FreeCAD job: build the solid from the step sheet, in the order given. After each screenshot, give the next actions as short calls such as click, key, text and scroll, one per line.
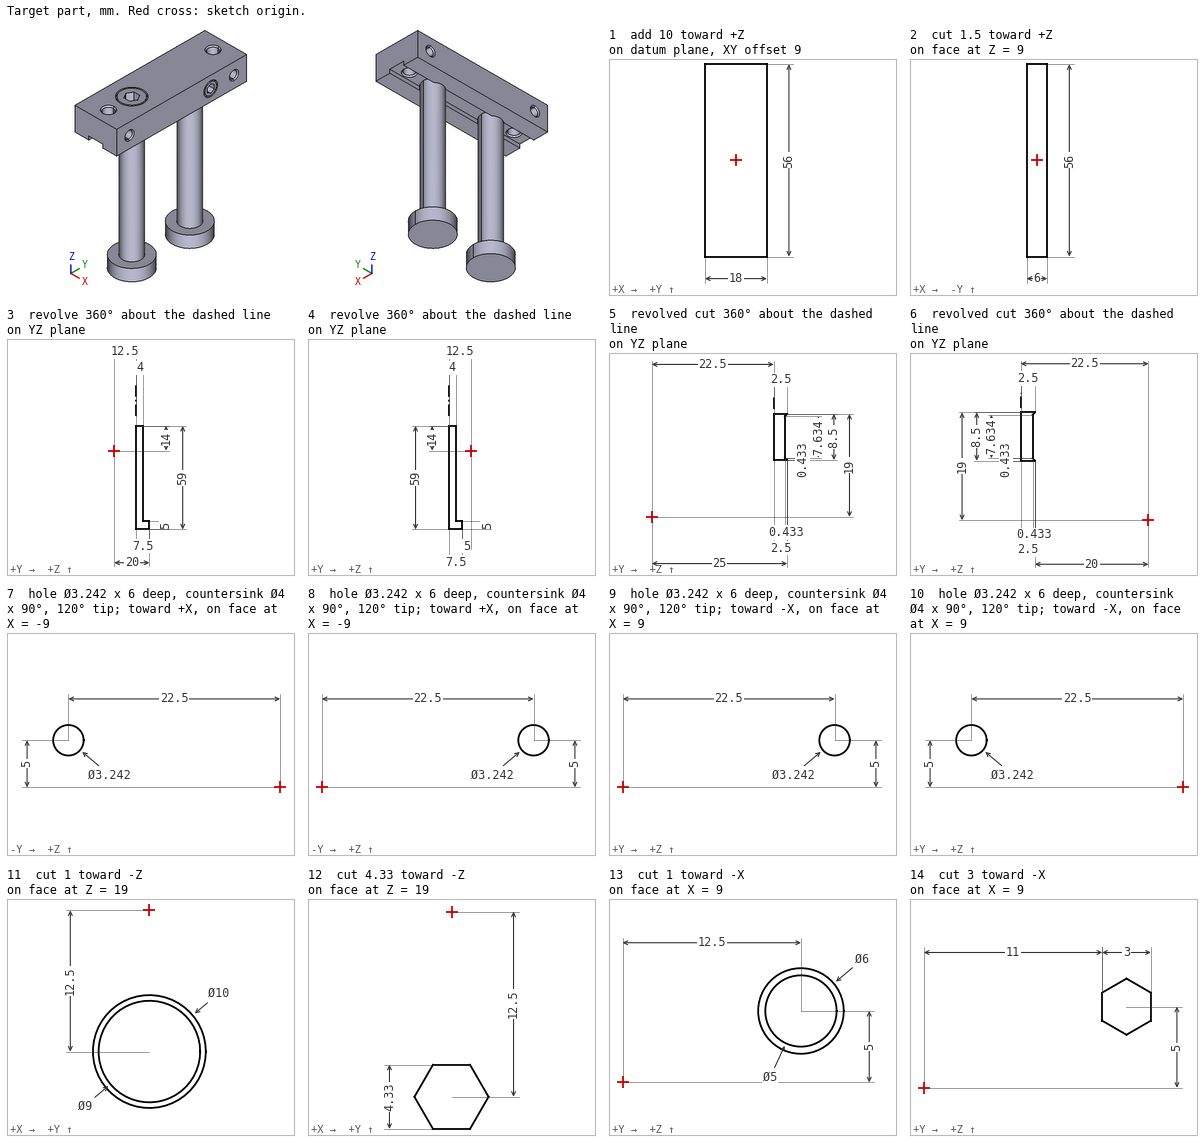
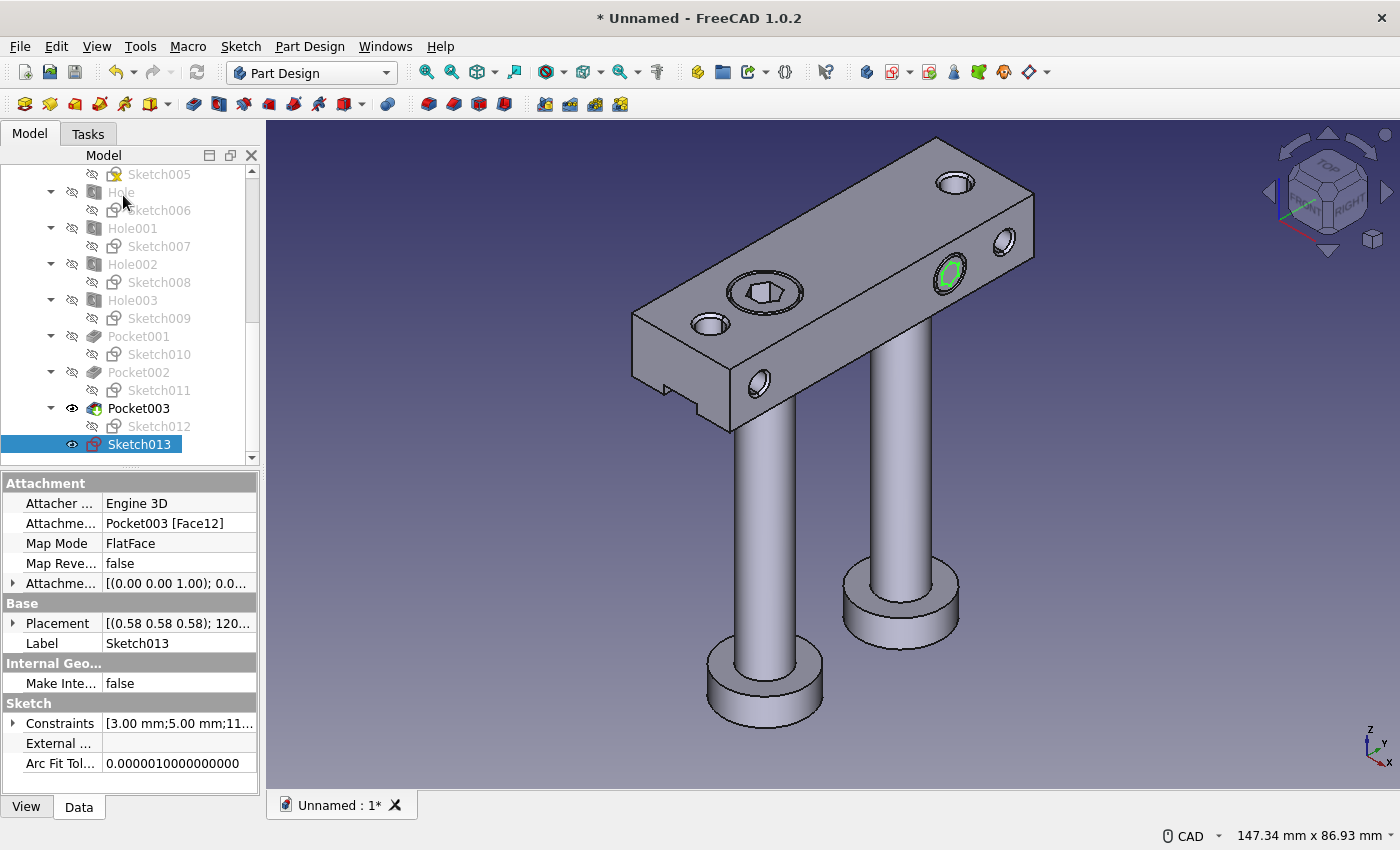
click(194, 104)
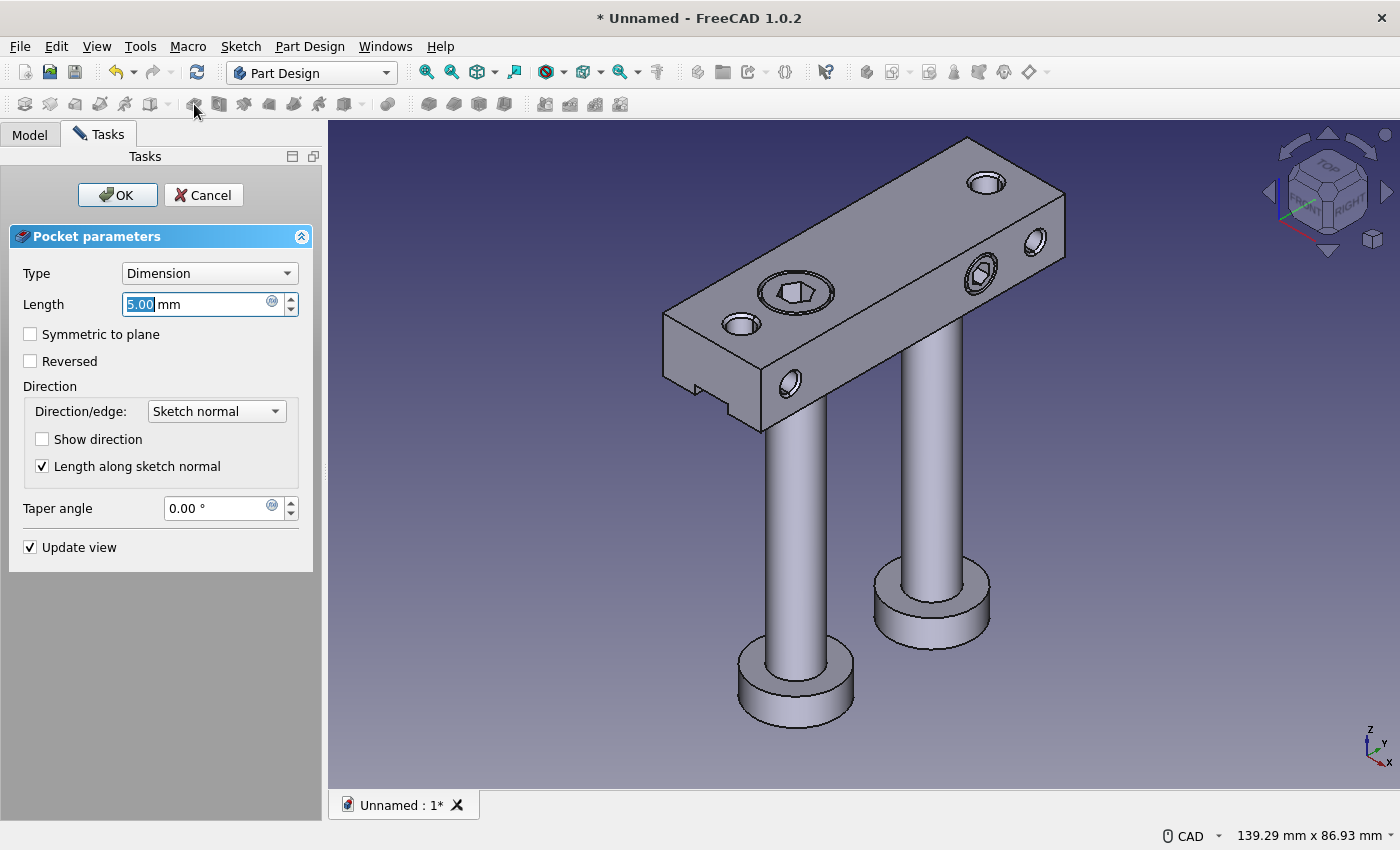
text(3)
key(Tab)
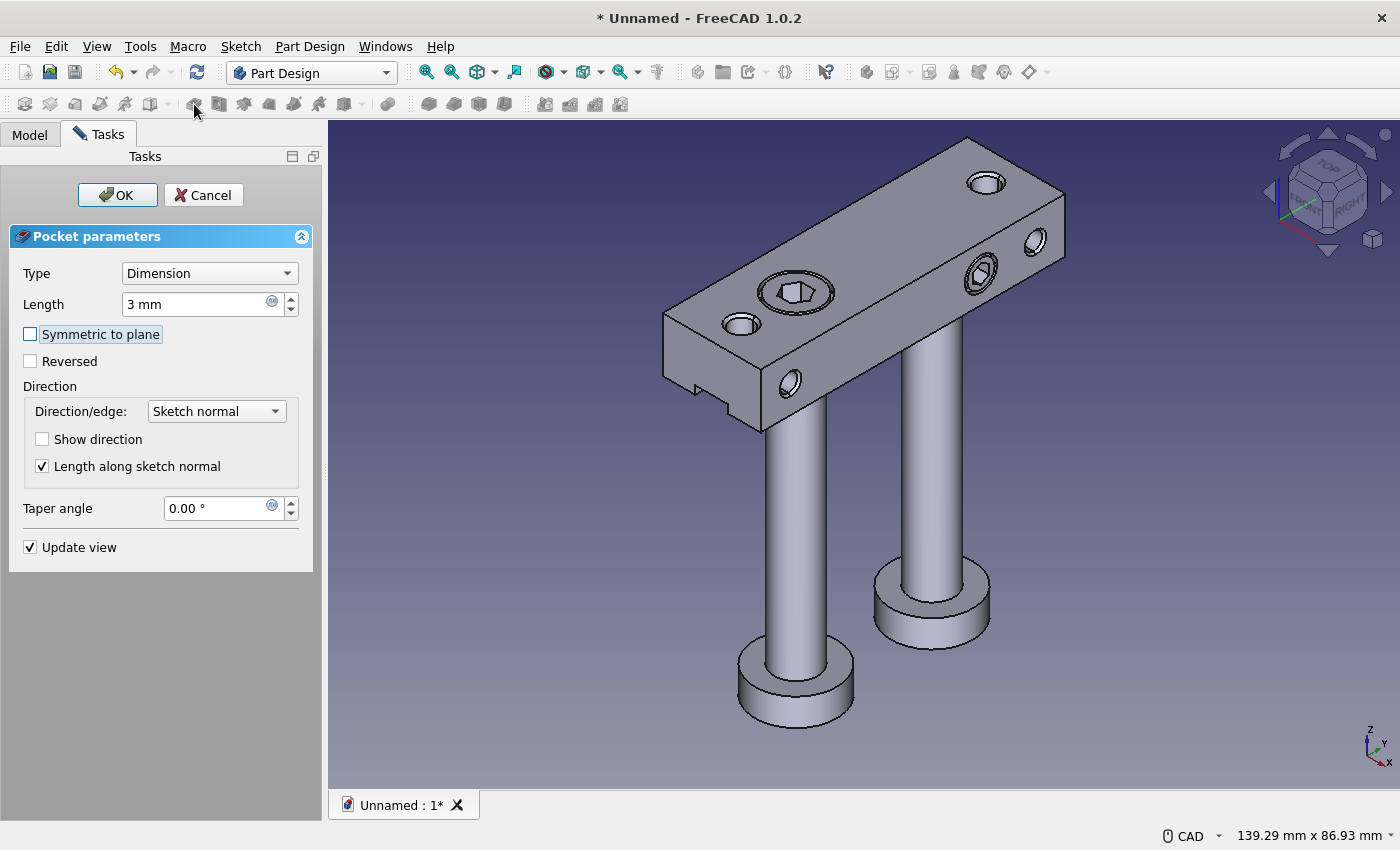
click(118, 195)